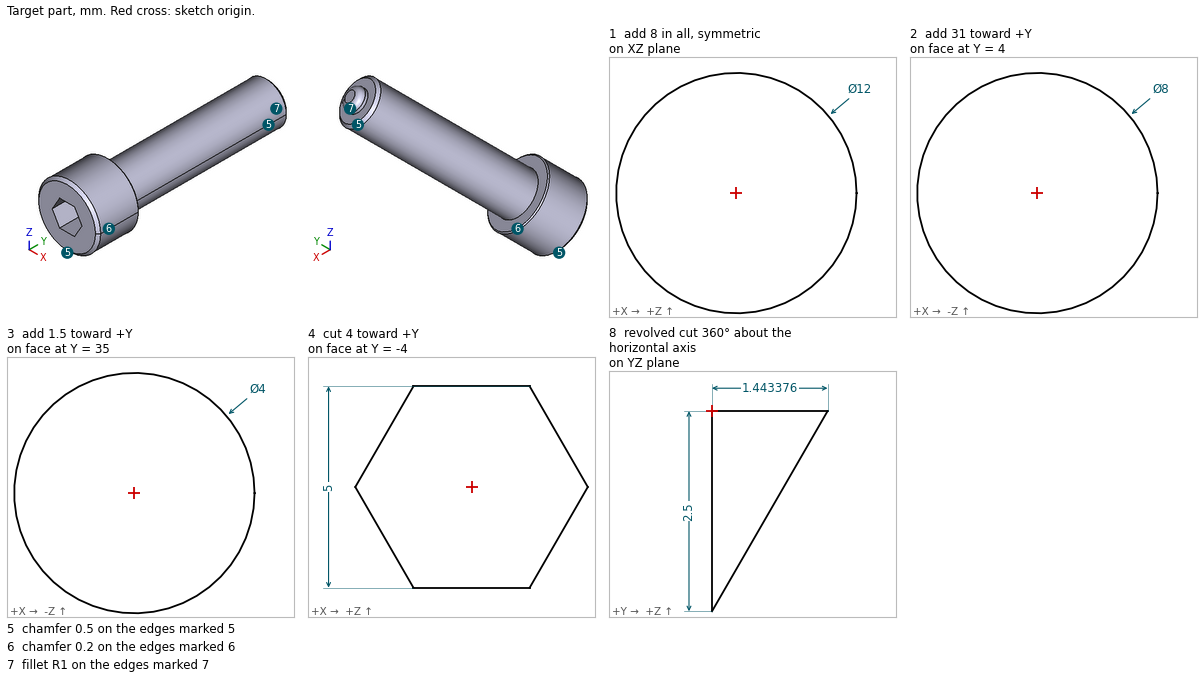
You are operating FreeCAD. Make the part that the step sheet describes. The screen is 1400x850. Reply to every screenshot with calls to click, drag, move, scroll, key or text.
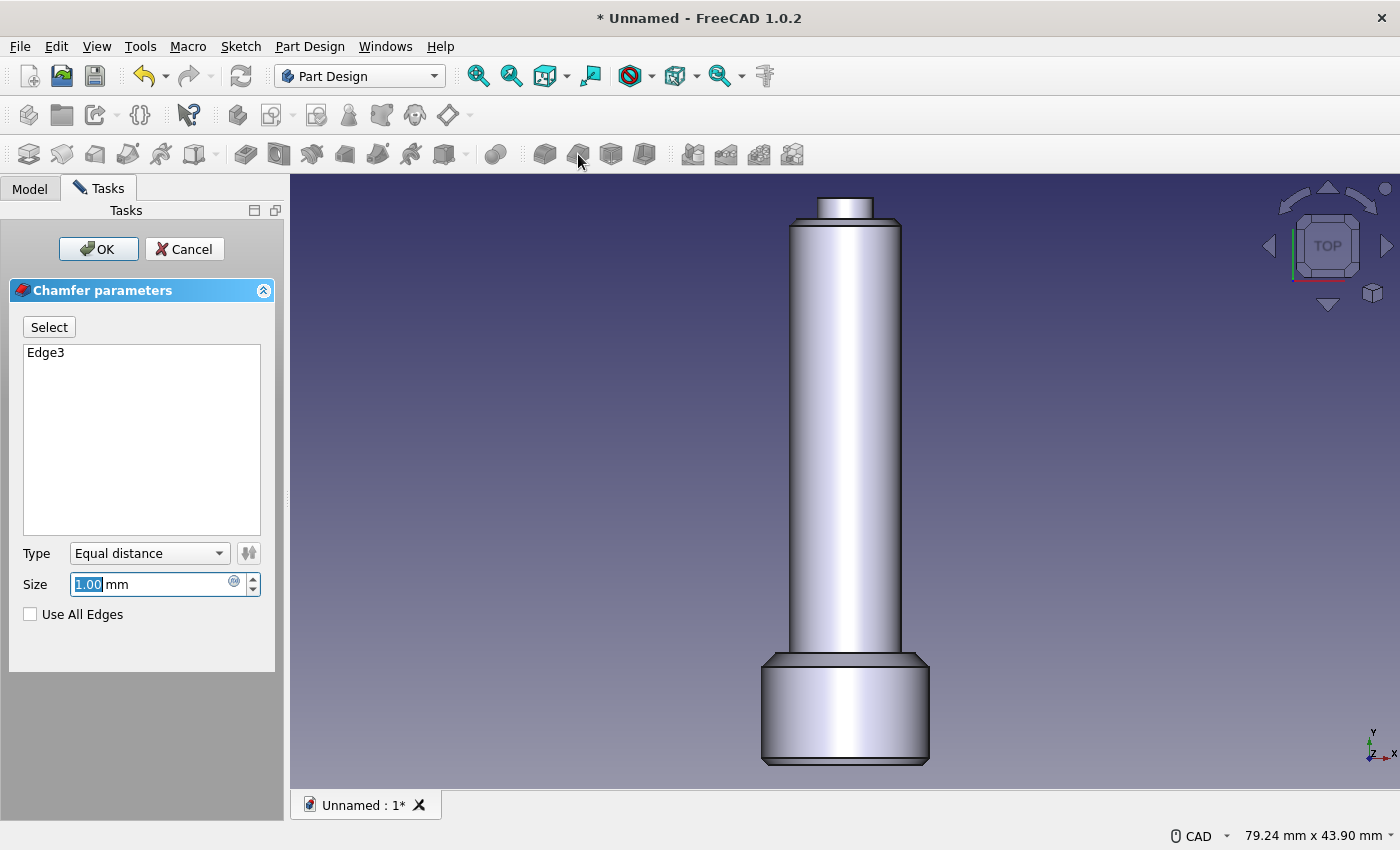
text(0.2)
key(Tab)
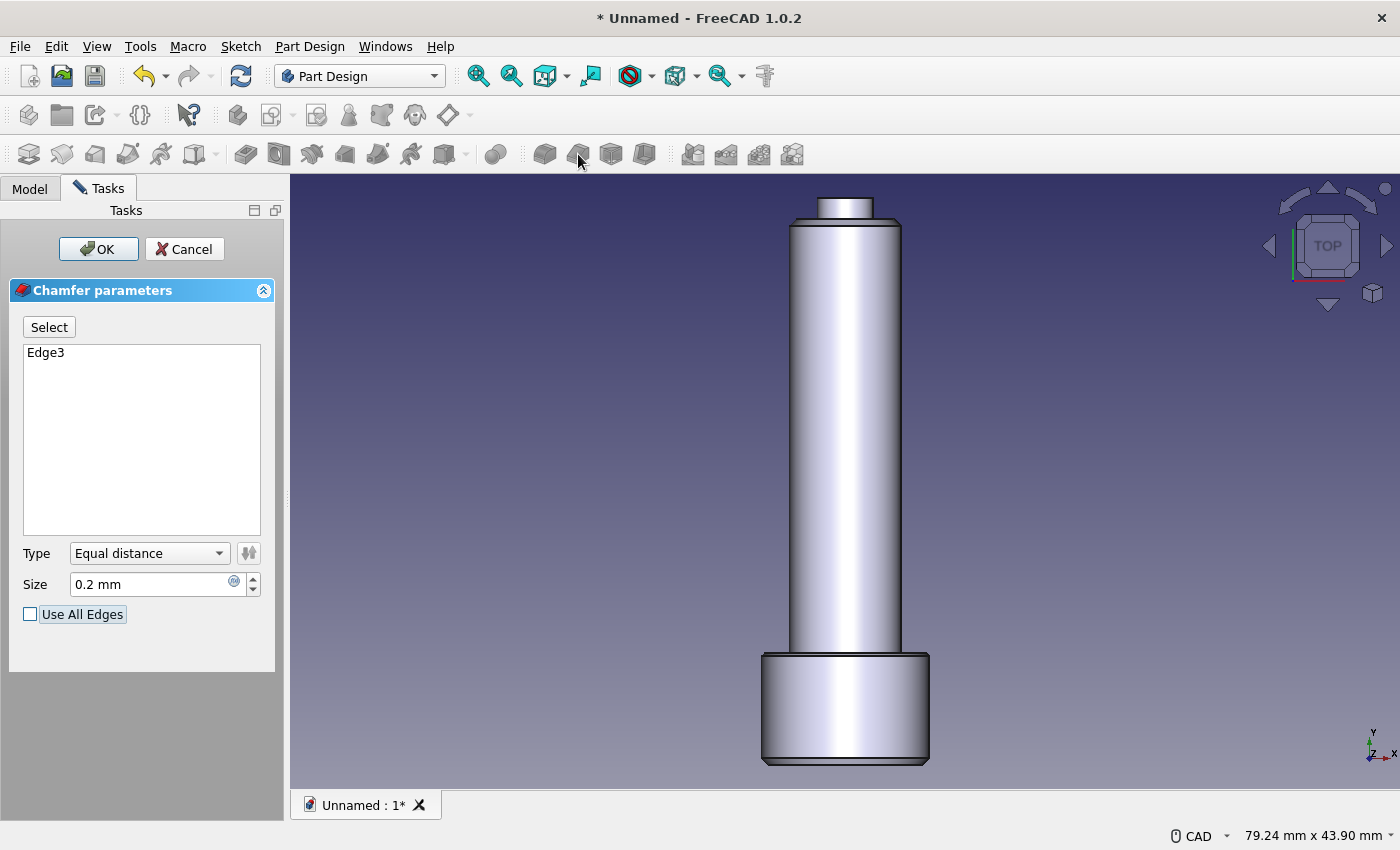
click(99, 249)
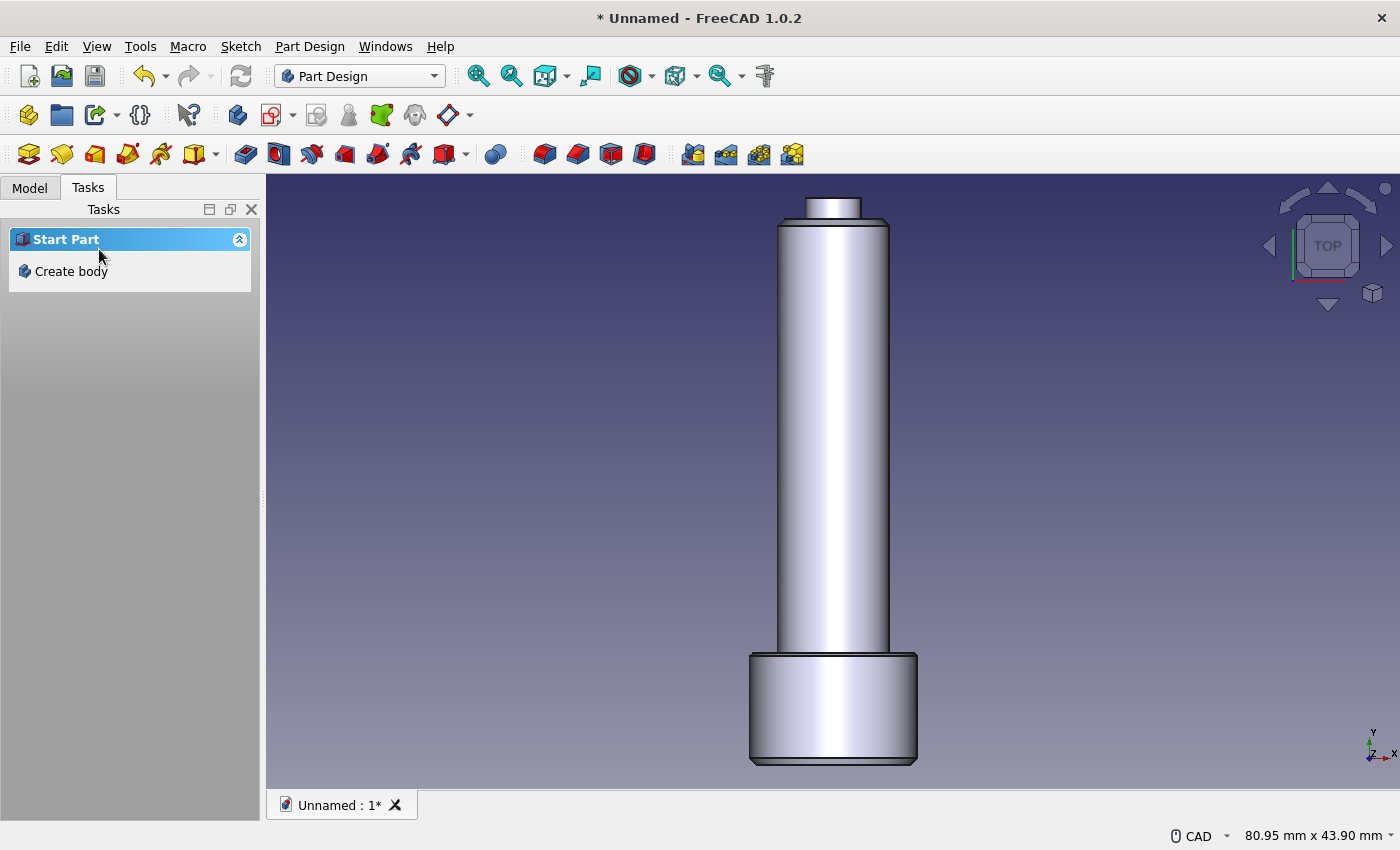
key(0)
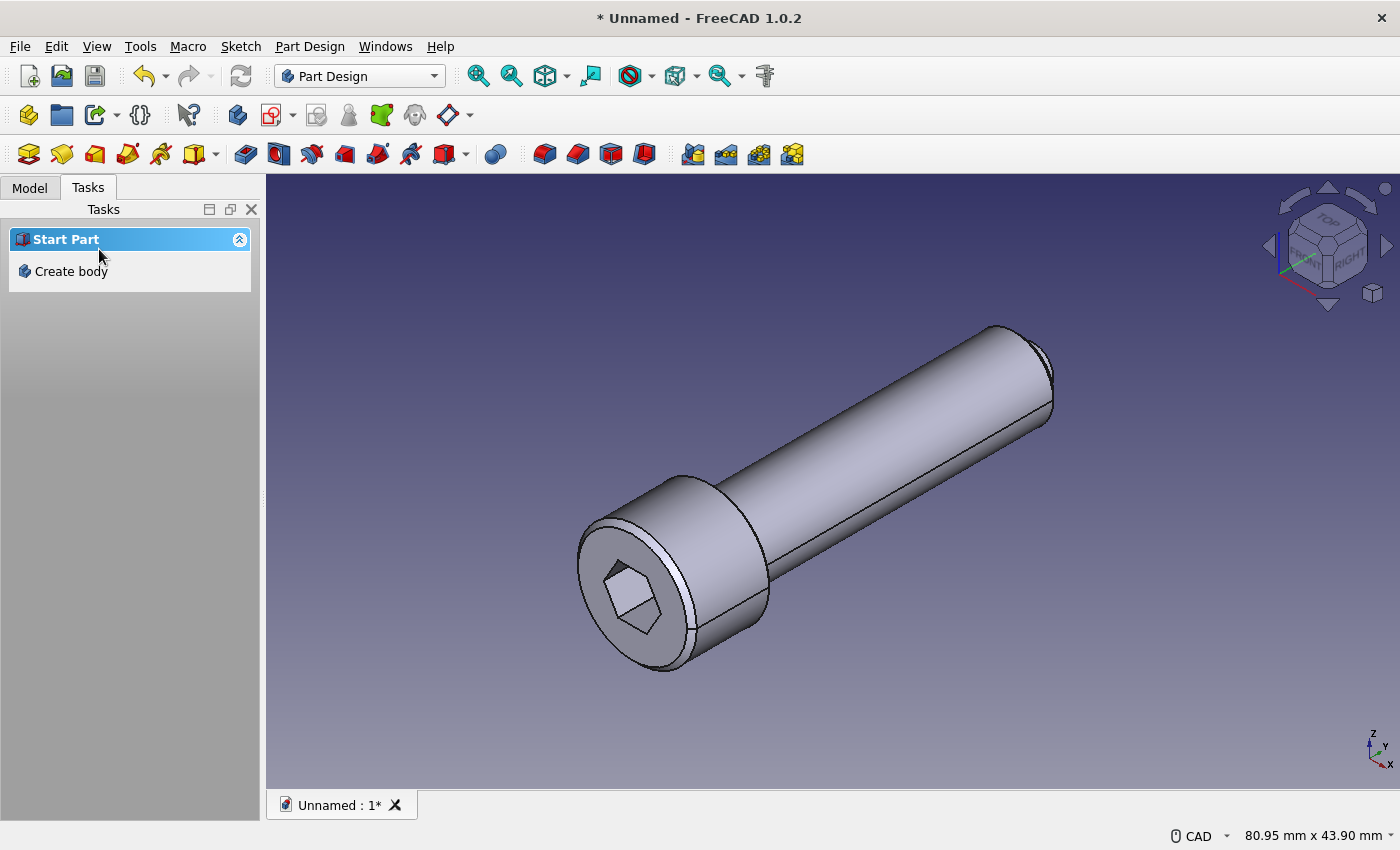
key(2)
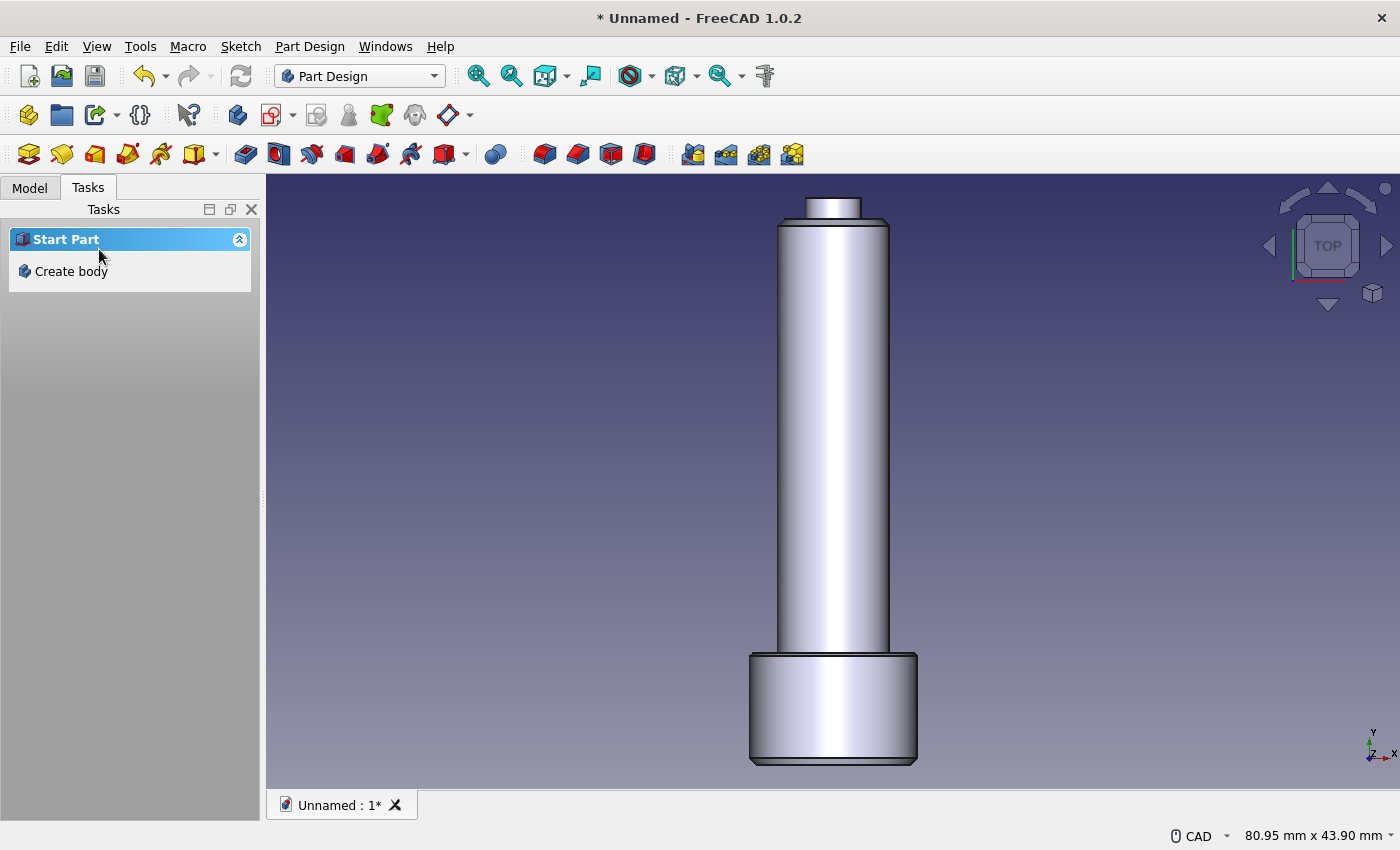
key(1)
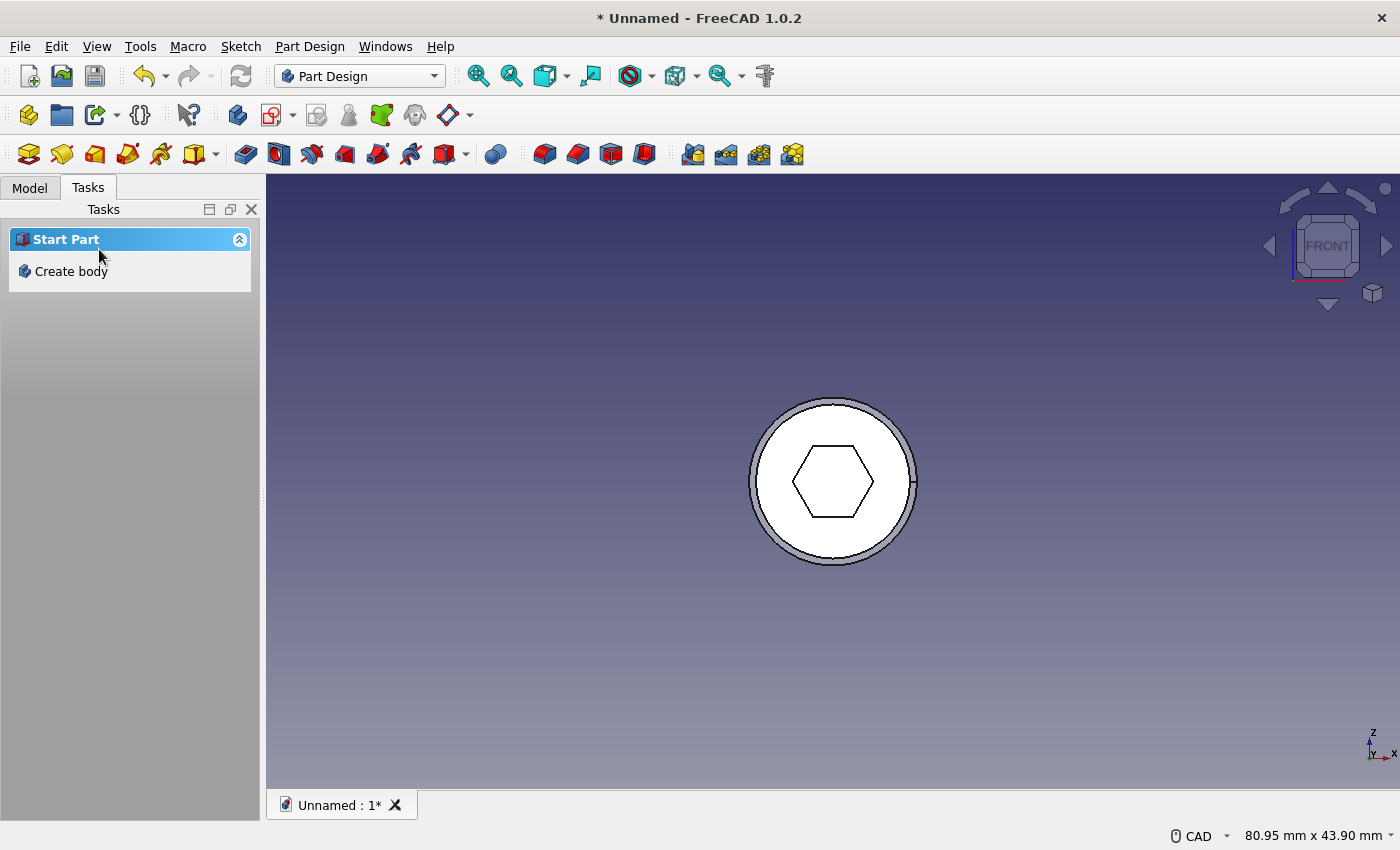
click(479, 76)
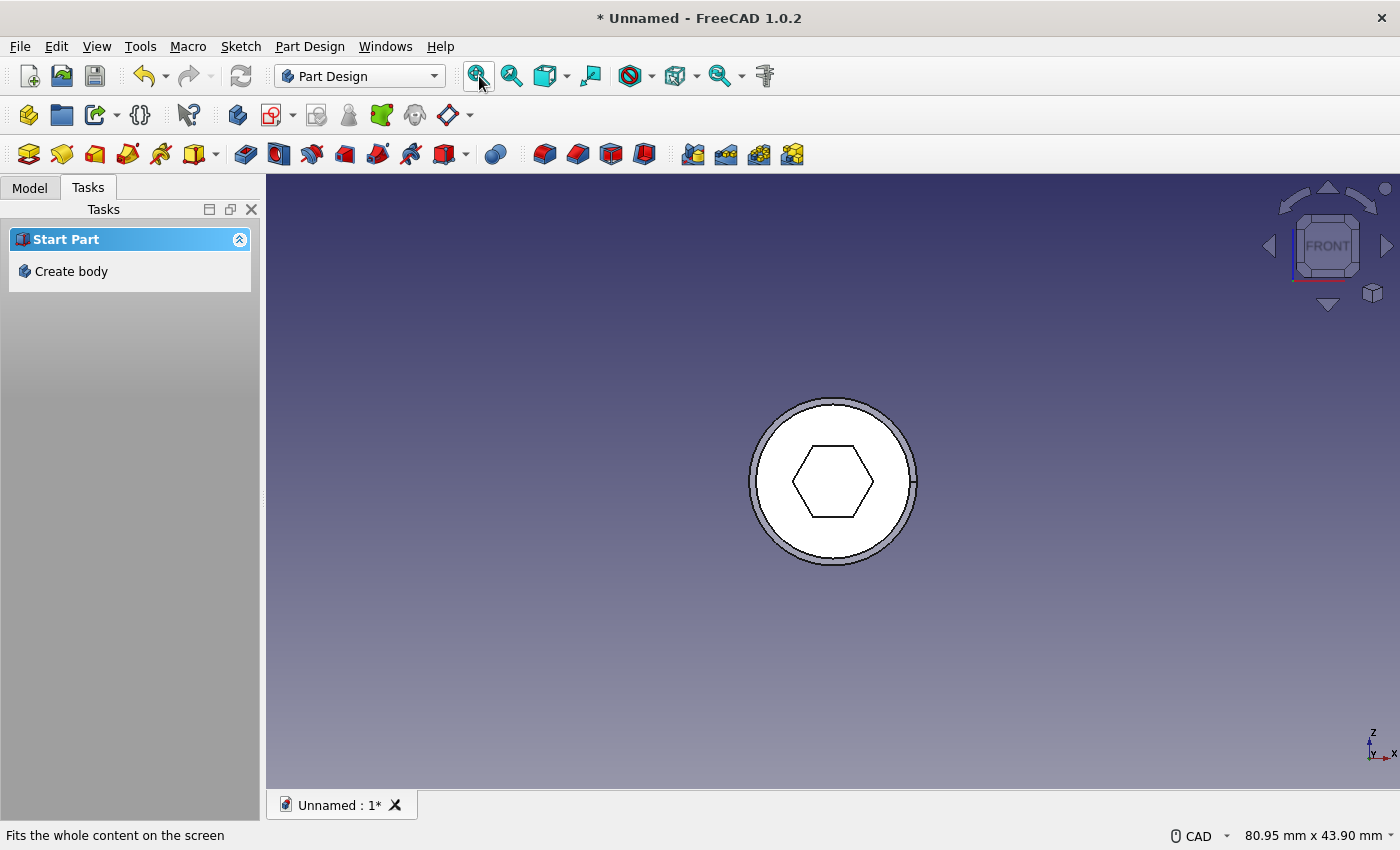
key(3)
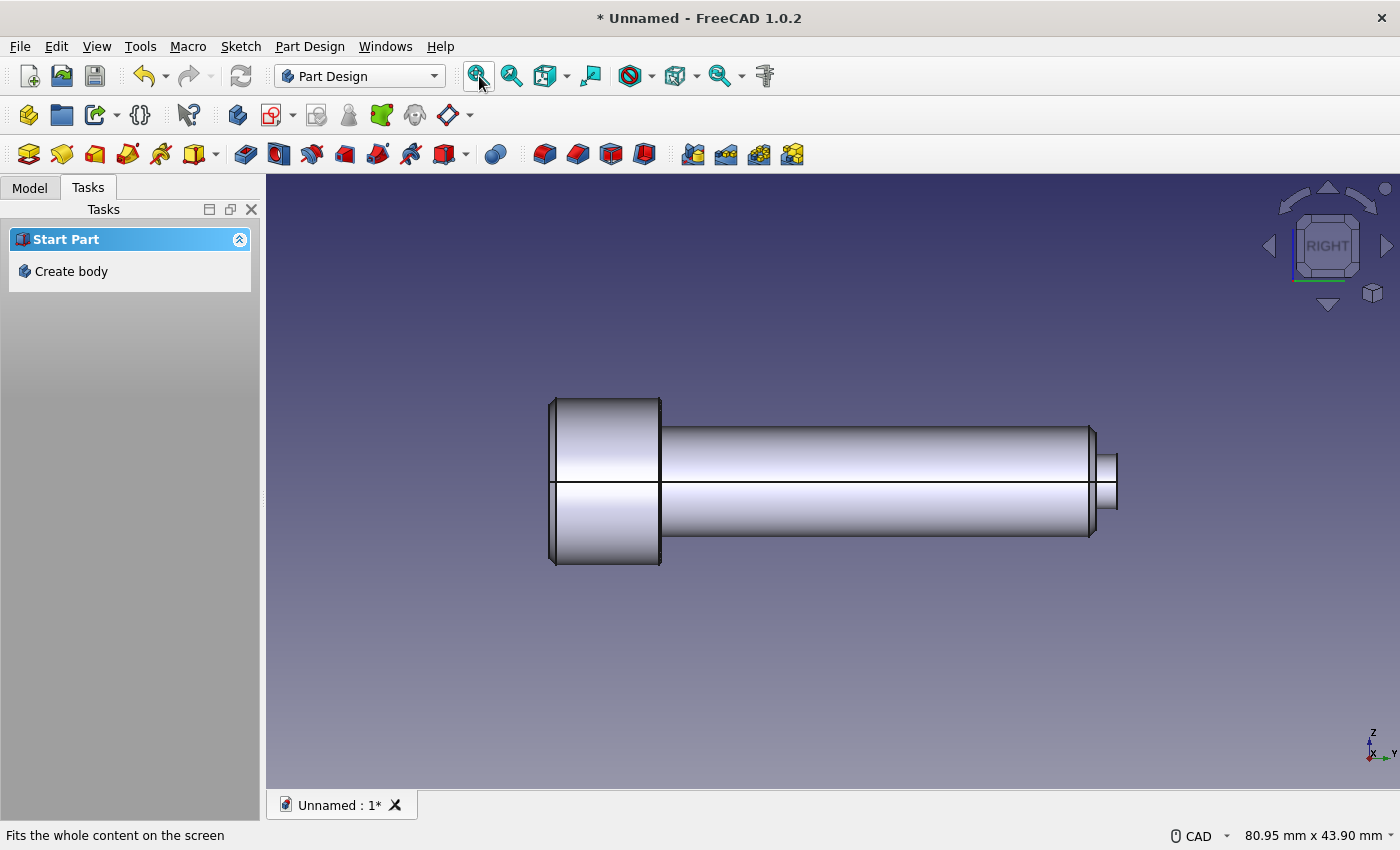
click(1117, 497)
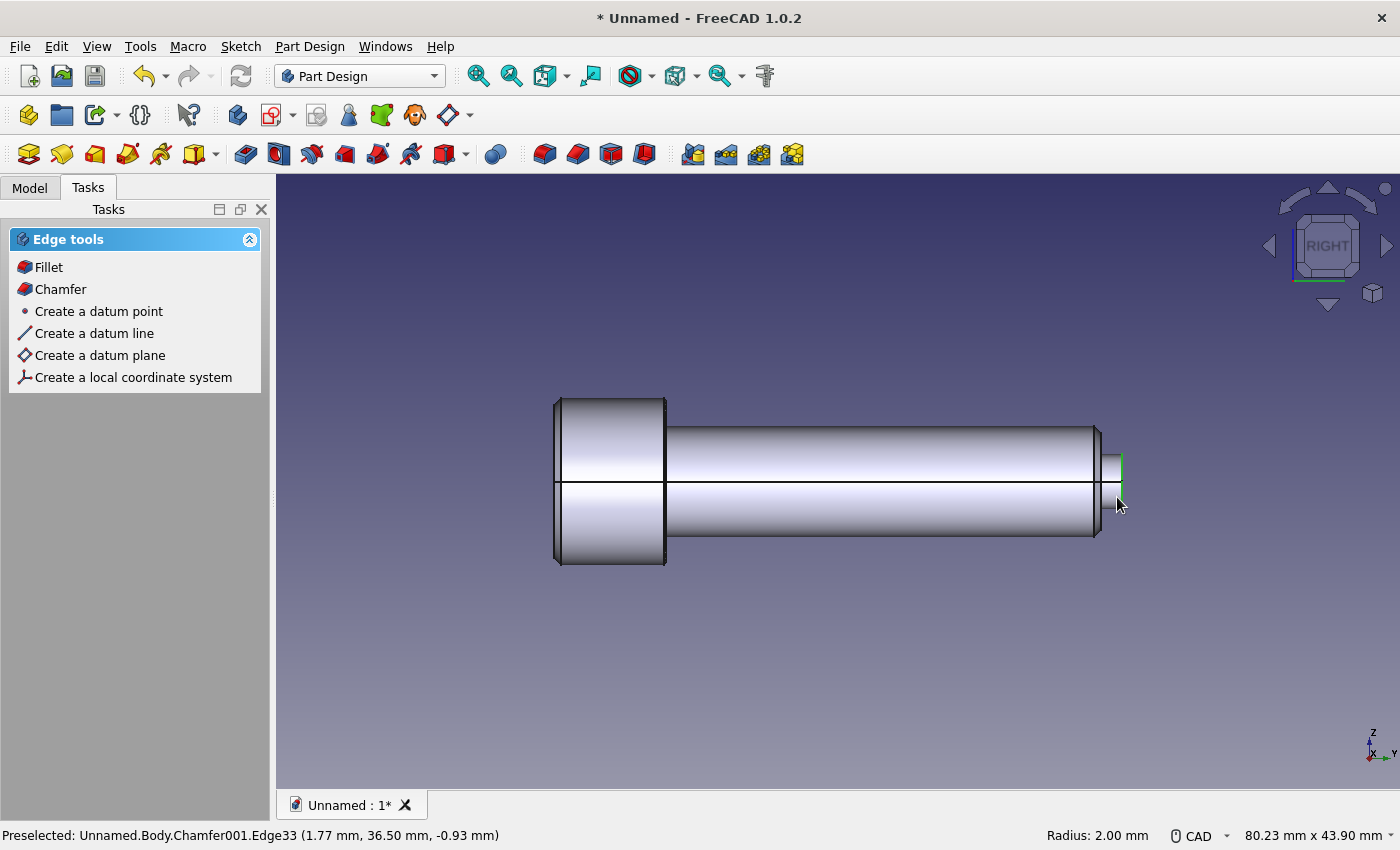
click(545, 154)